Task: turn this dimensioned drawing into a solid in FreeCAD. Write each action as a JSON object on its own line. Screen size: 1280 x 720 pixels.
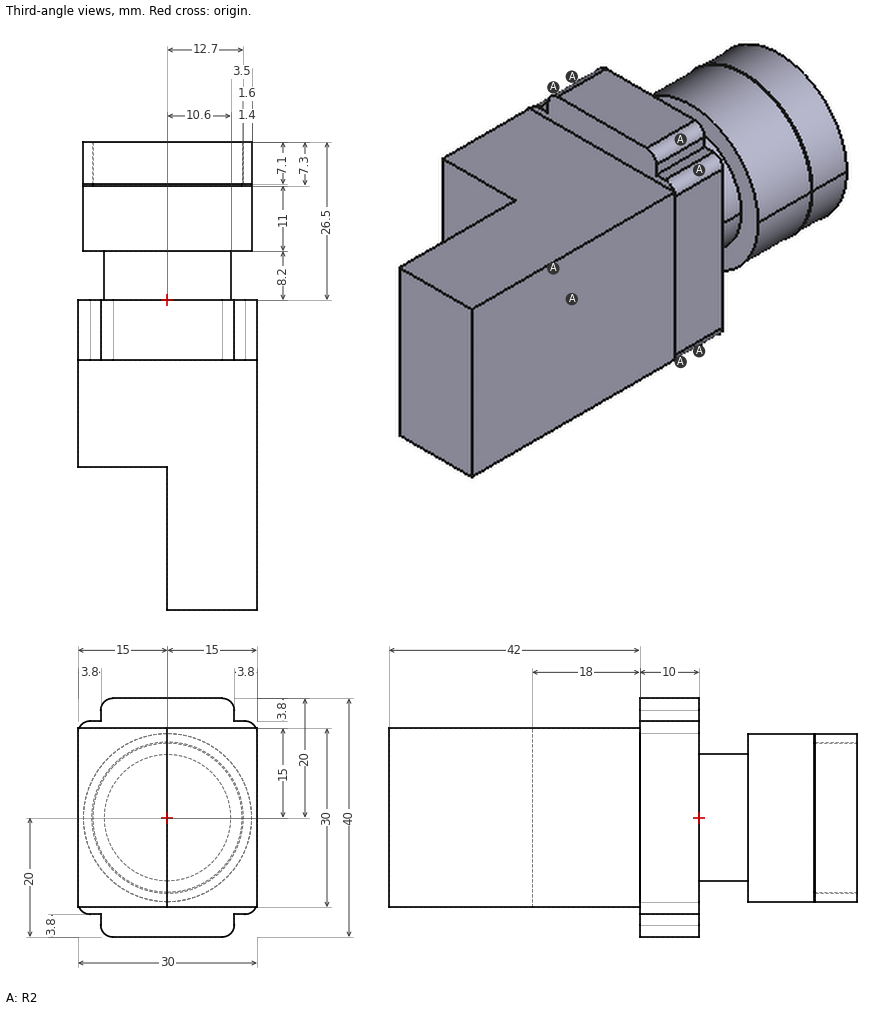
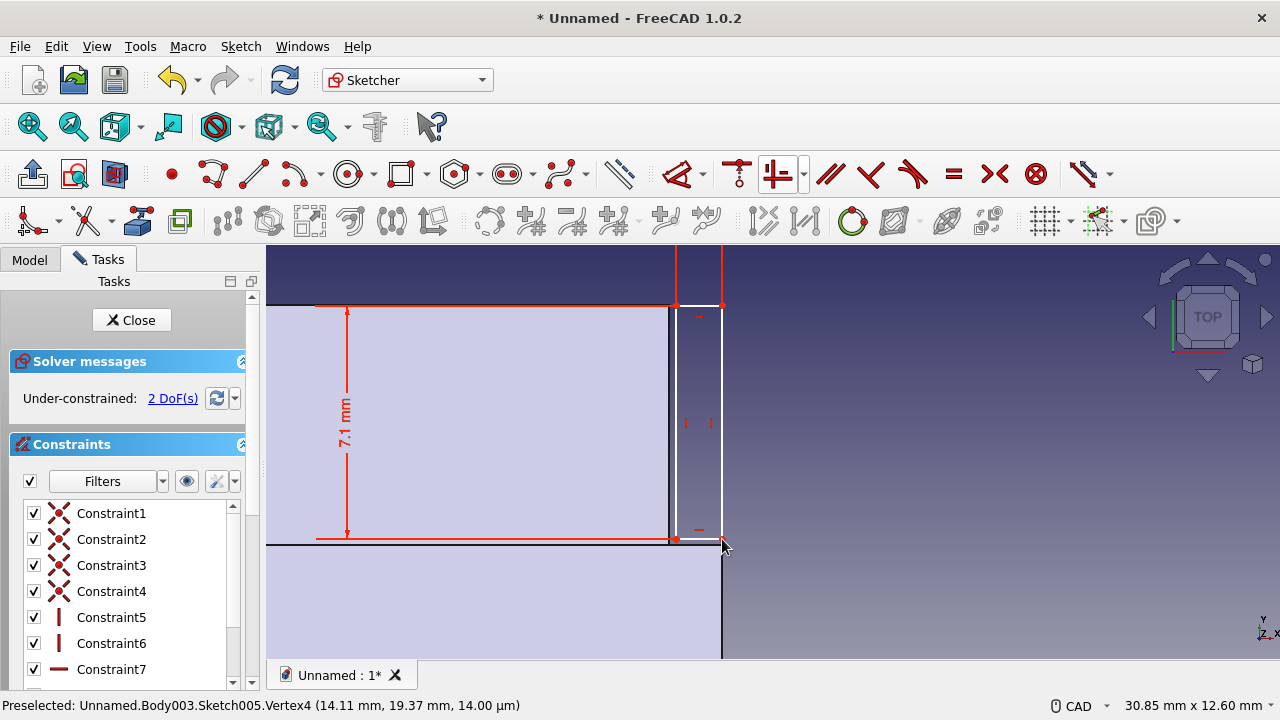
{"action": "key", "text": "d"}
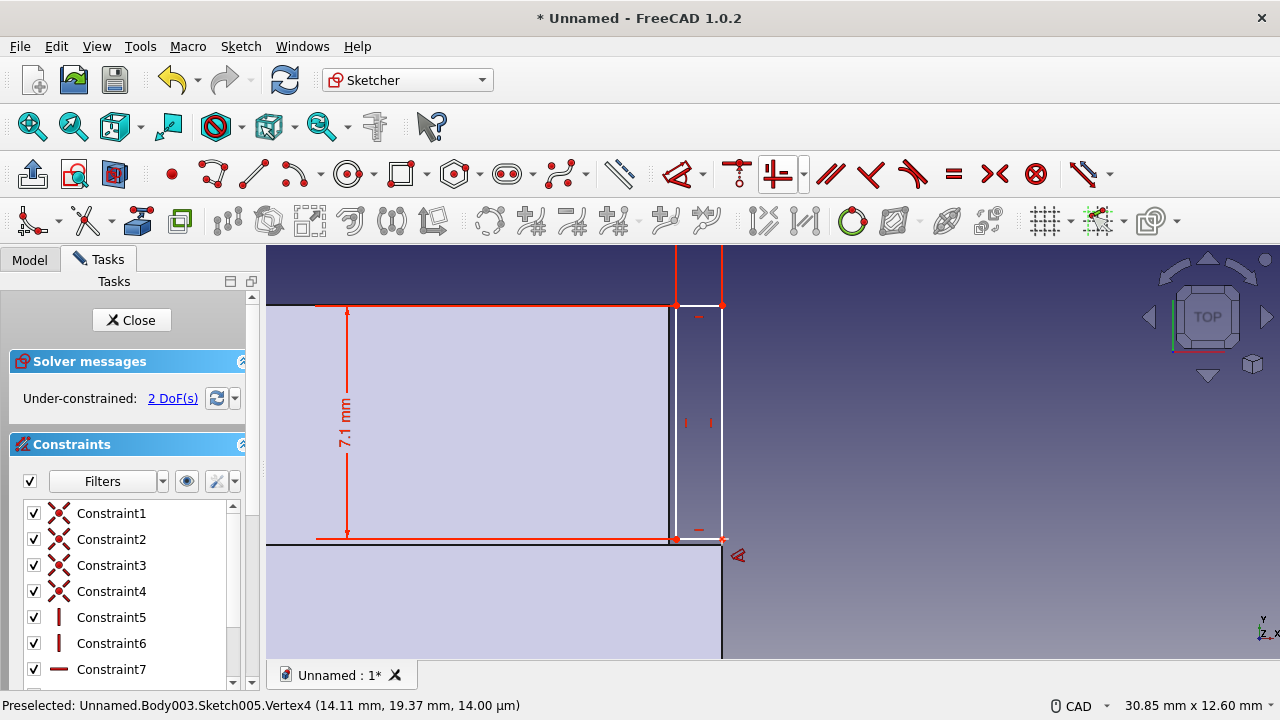
{"action": "left_click", "coordinate": [676, 306]}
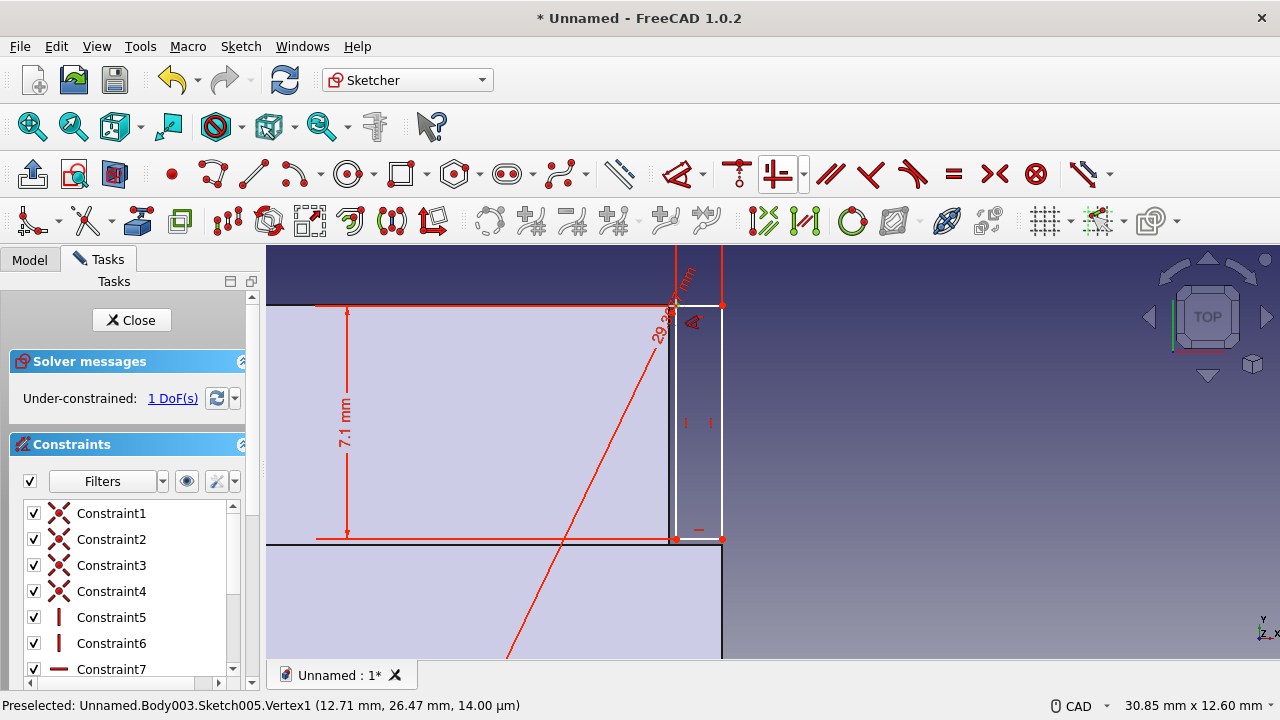
{"action": "key", "text": "Escape"}
{"action": "key", "text": "Escape"}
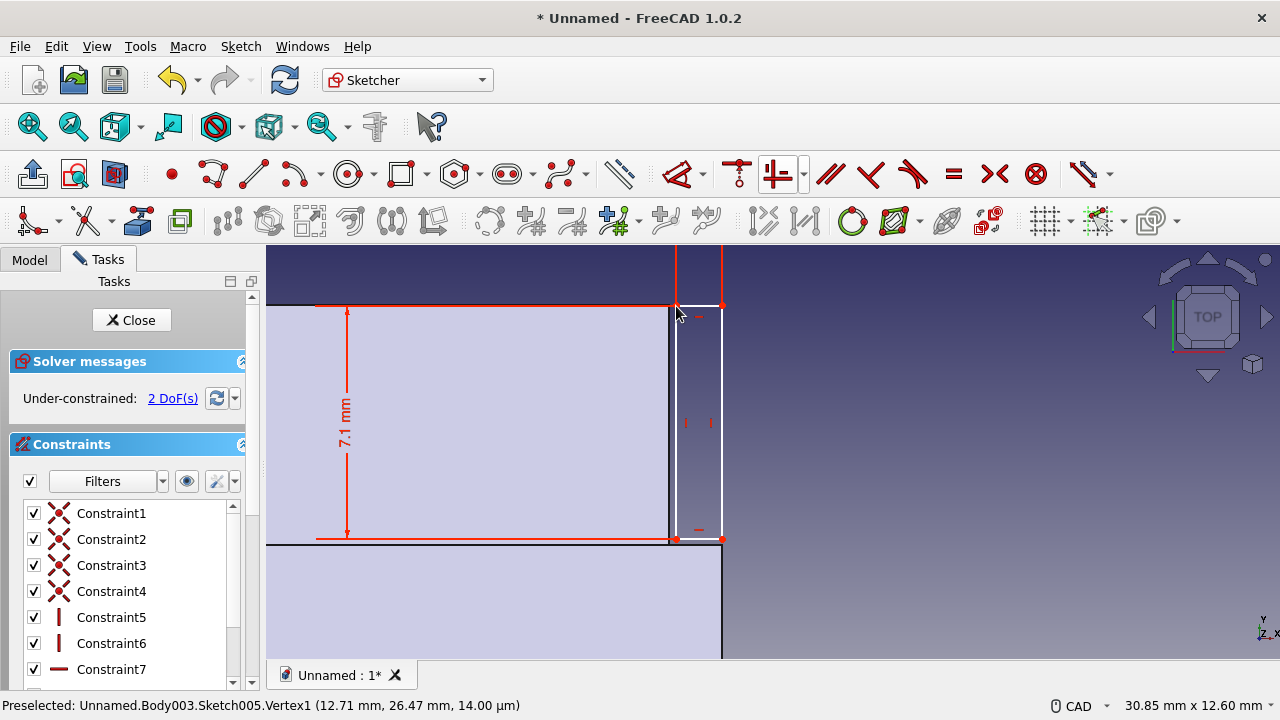
{"action": "left_click", "coordinate": [676, 306]}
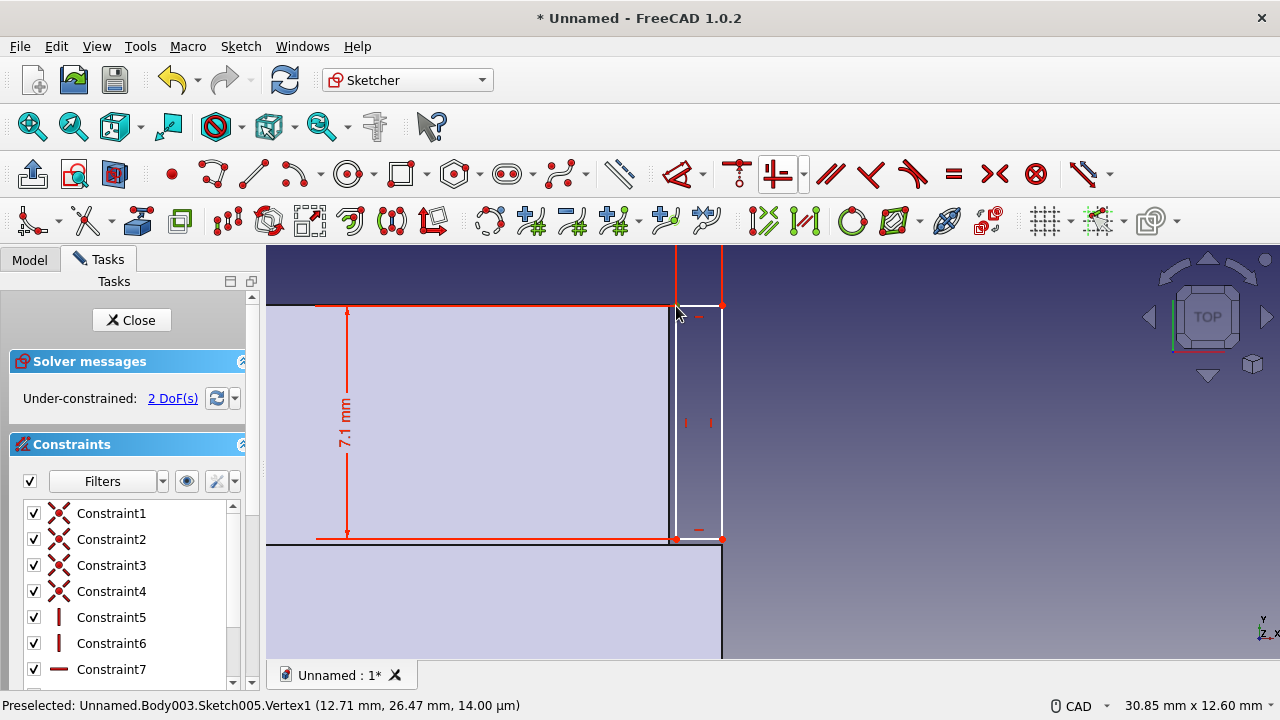
{"action": "key", "text": "l"}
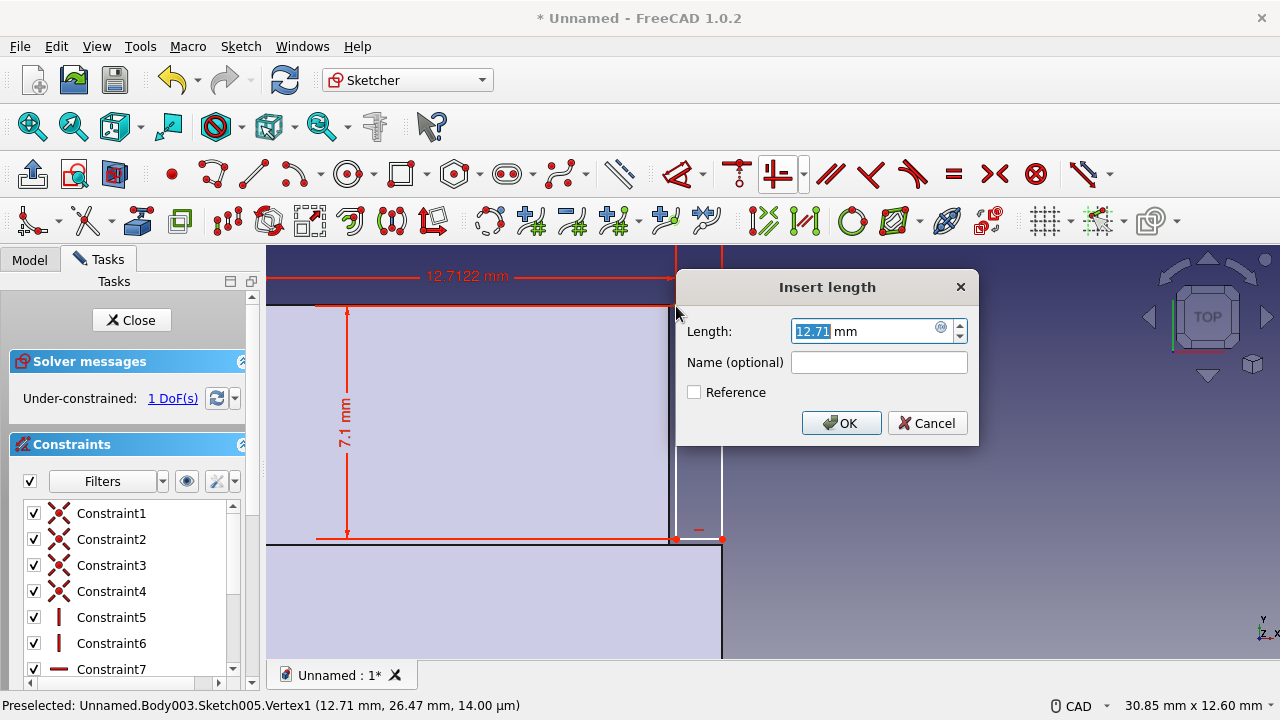
{"action": "type", "text": "12.7"}
{"action": "key", "text": "Return"}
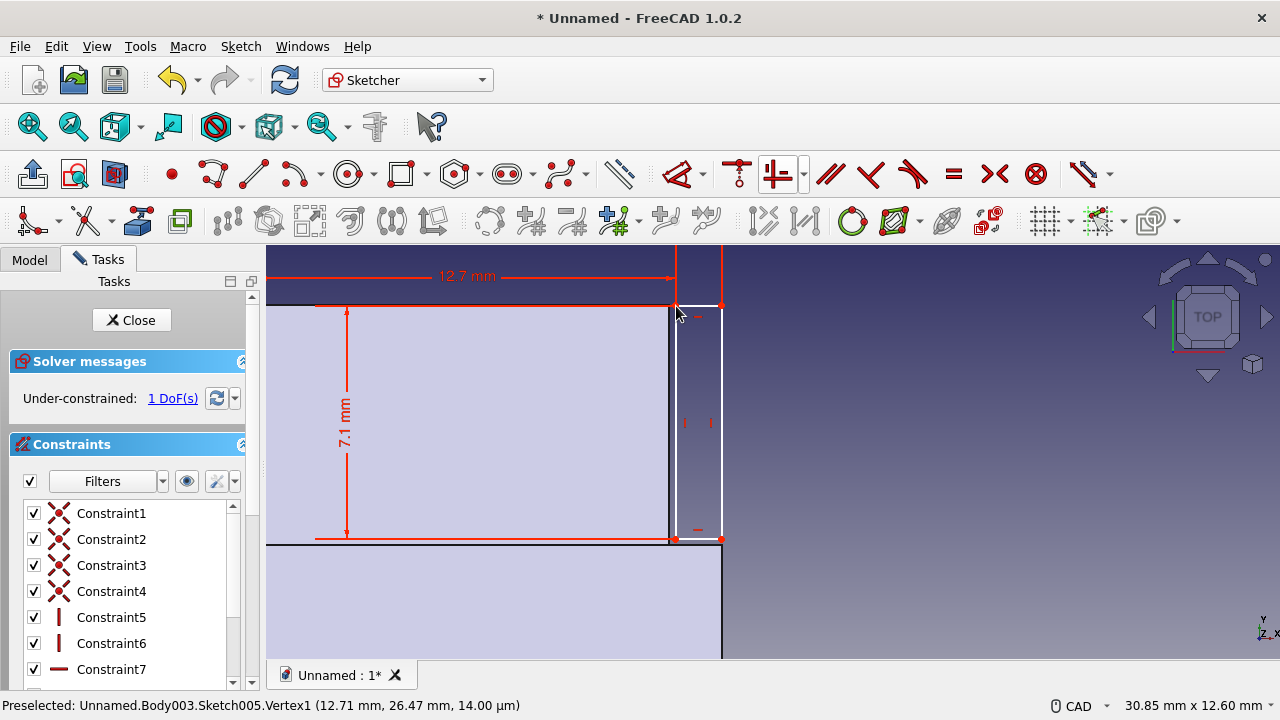
{"action": "left_click", "coordinate": [676, 306]}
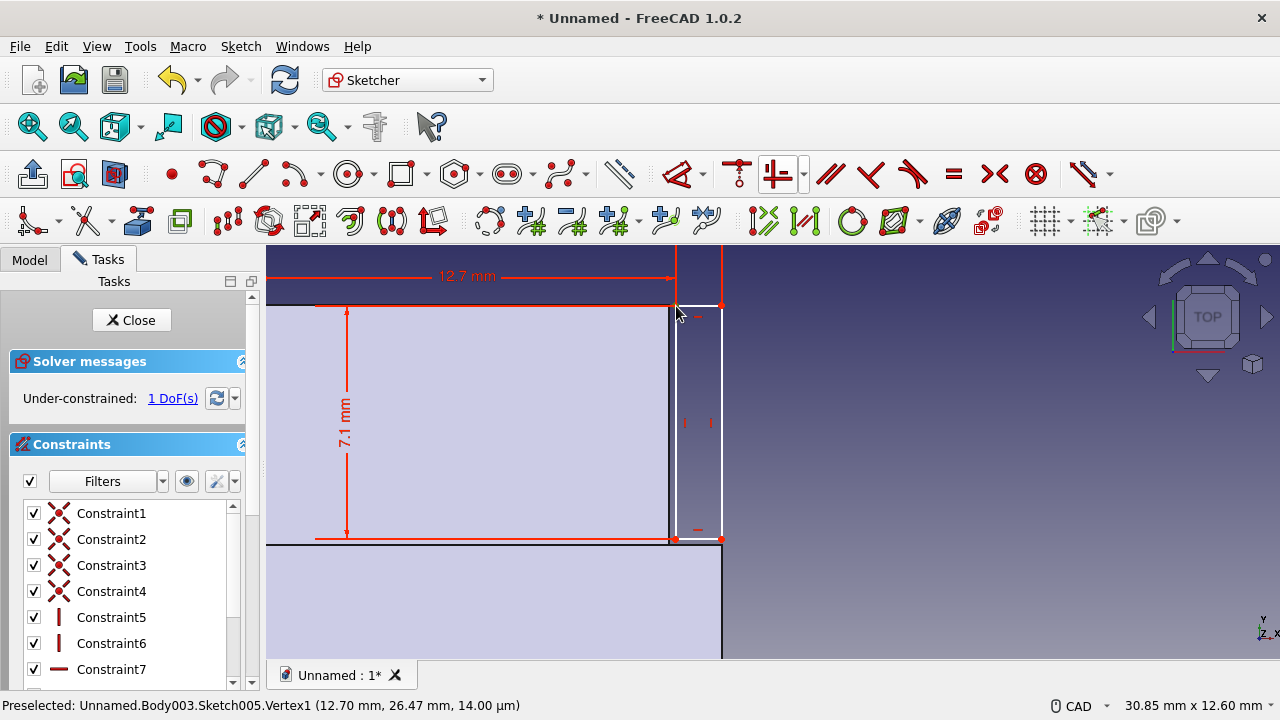
{"action": "key", "text": "i"}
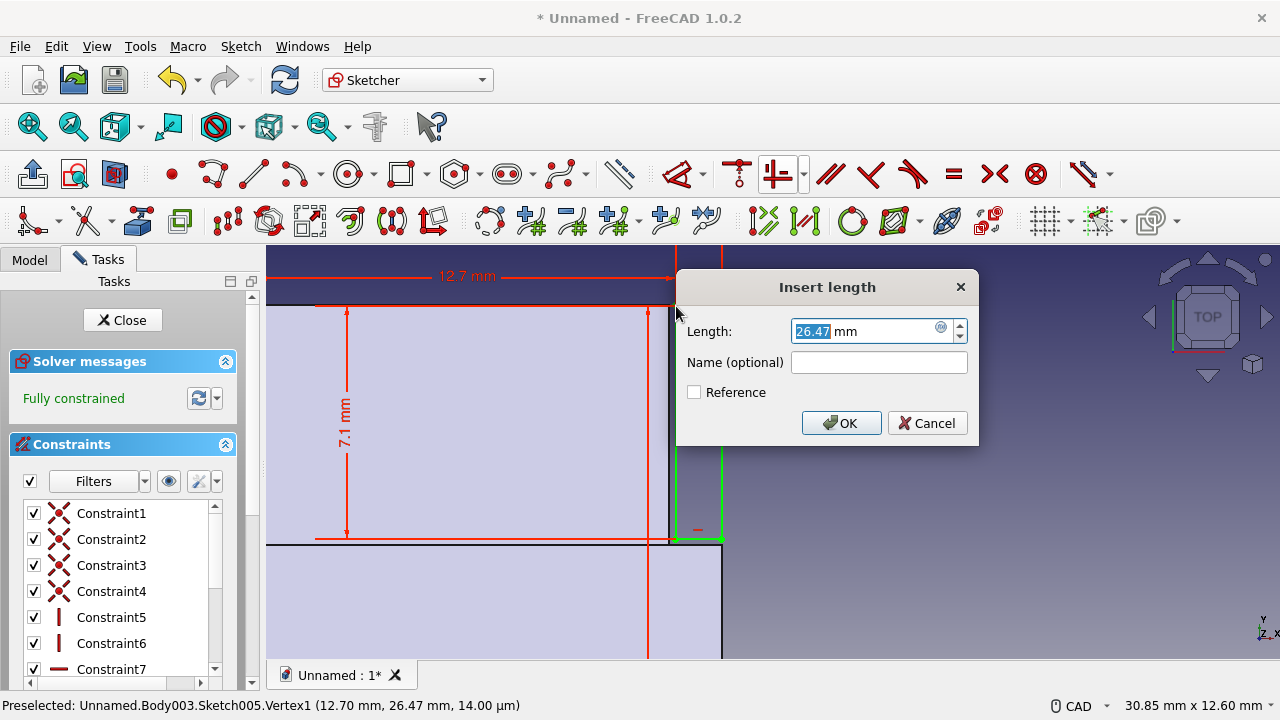
{"action": "type", "text": "26.5"}
{"action": "key", "text": "Return"}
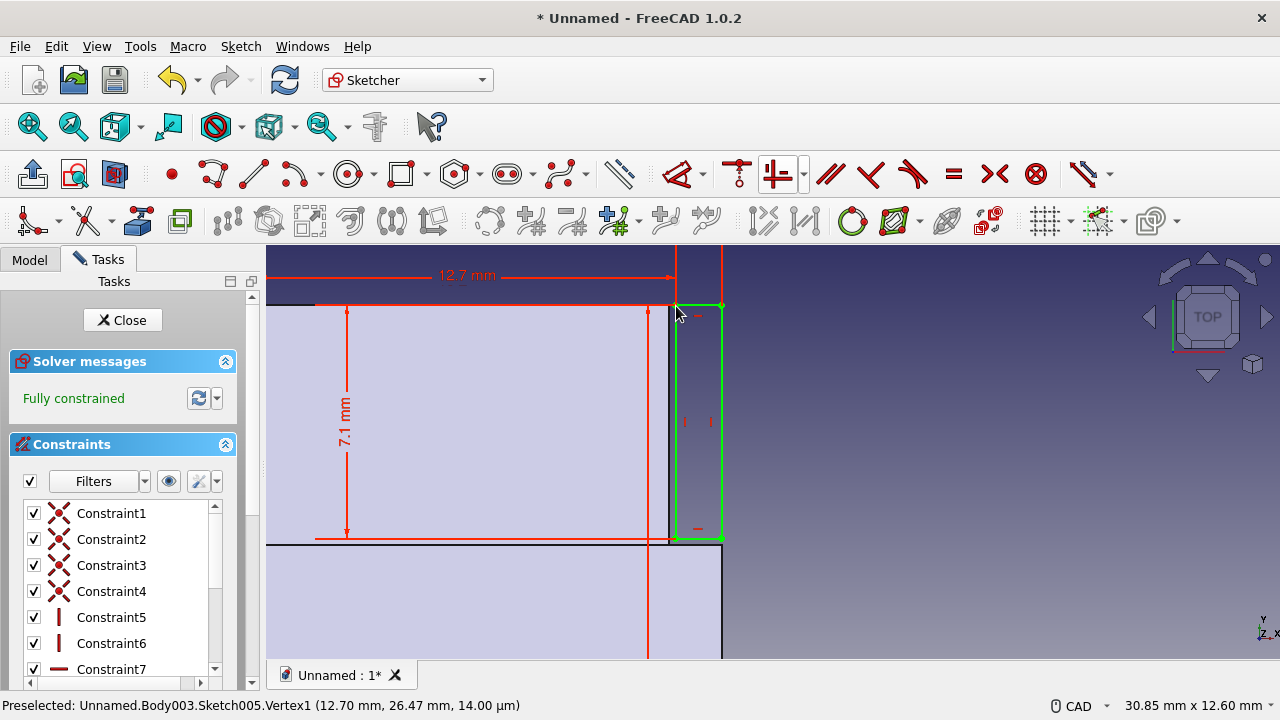
{"action": "left_click", "coordinate": [123, 320]}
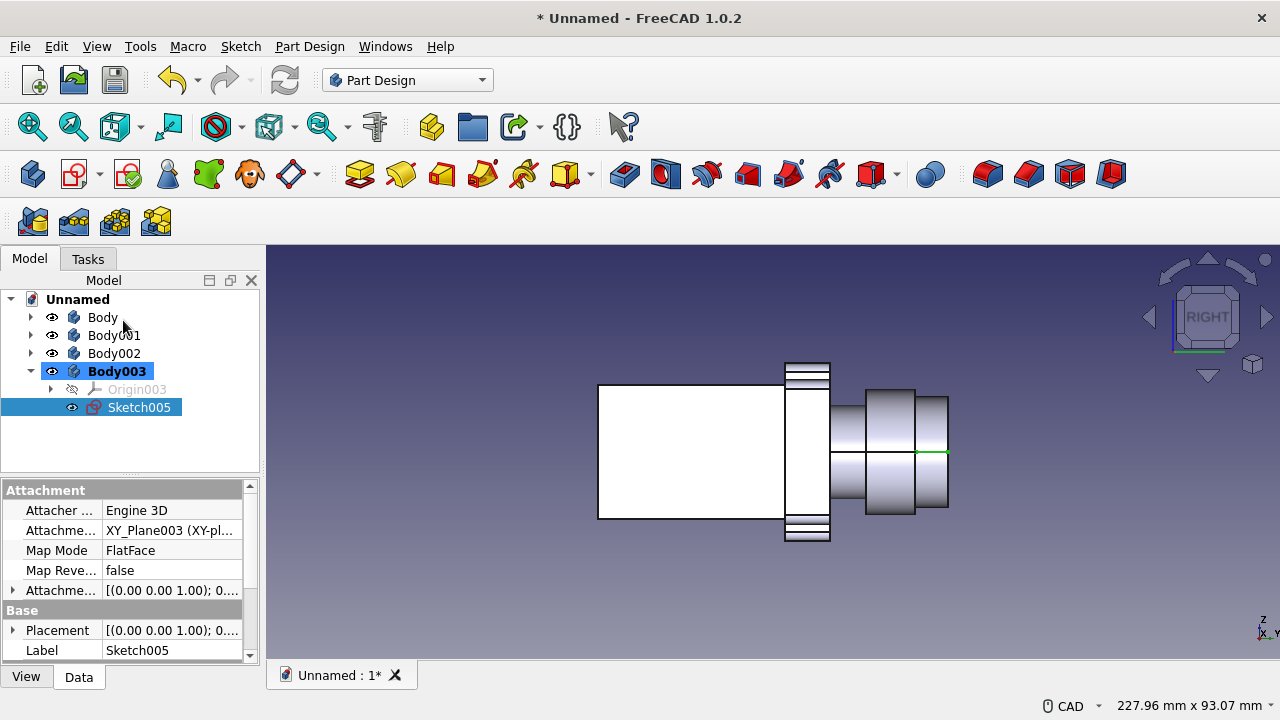
{"action": "left_click", "coordinate": [401, 174]}